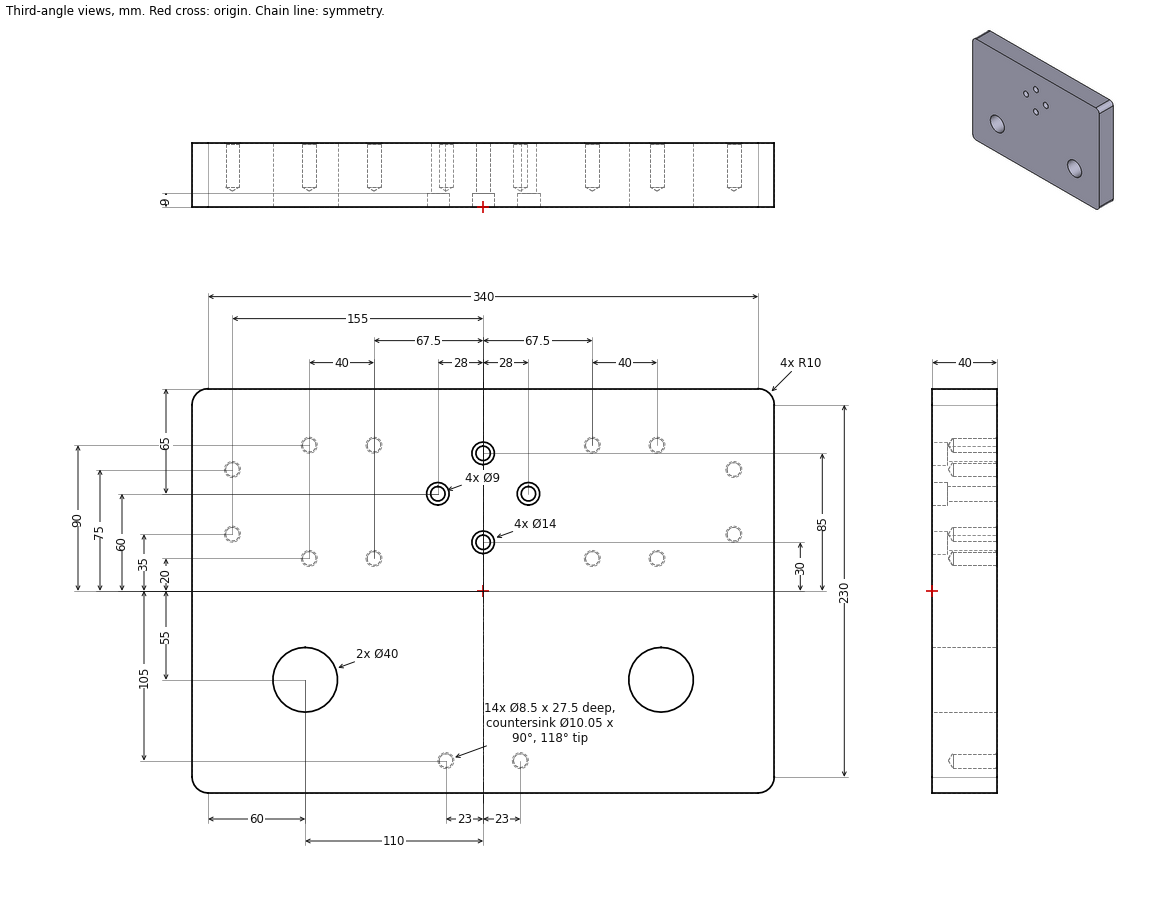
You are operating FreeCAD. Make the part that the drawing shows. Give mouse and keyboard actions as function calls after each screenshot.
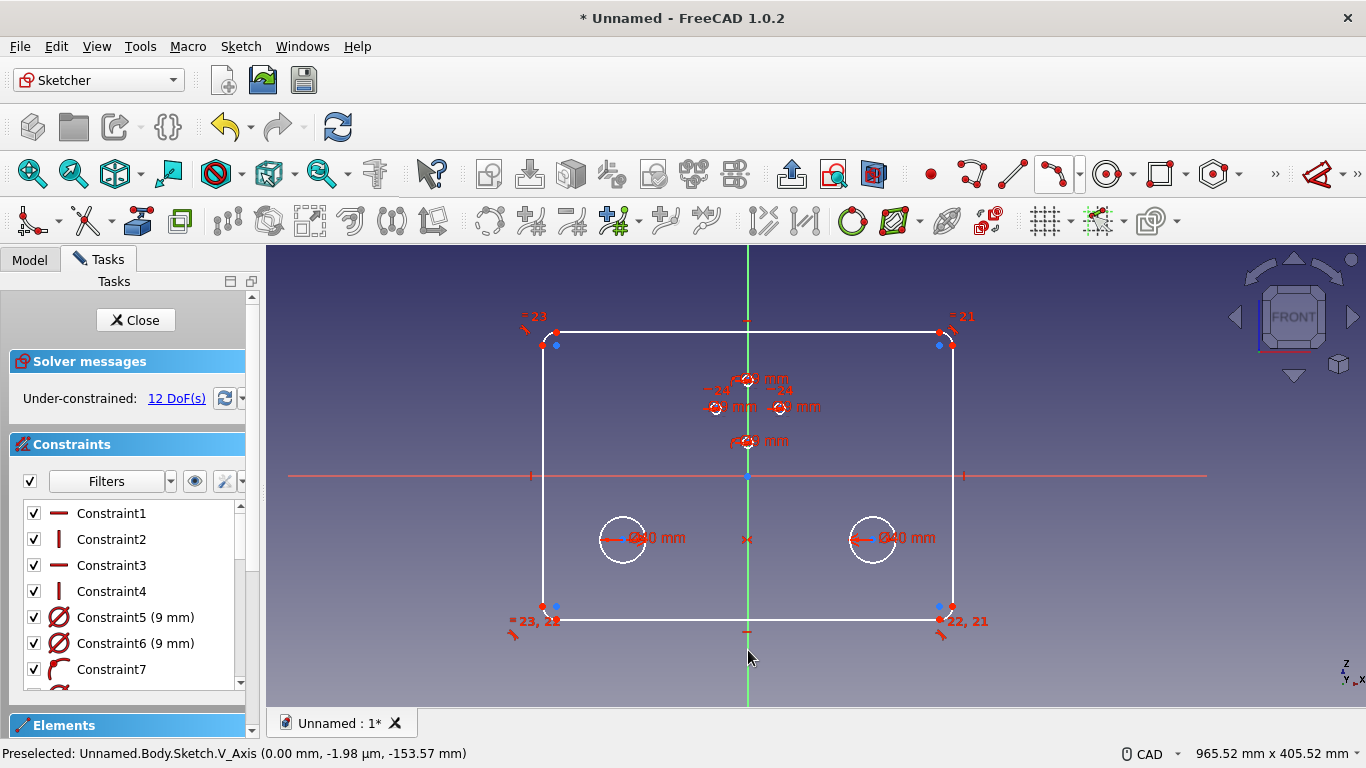
click(1316, 174)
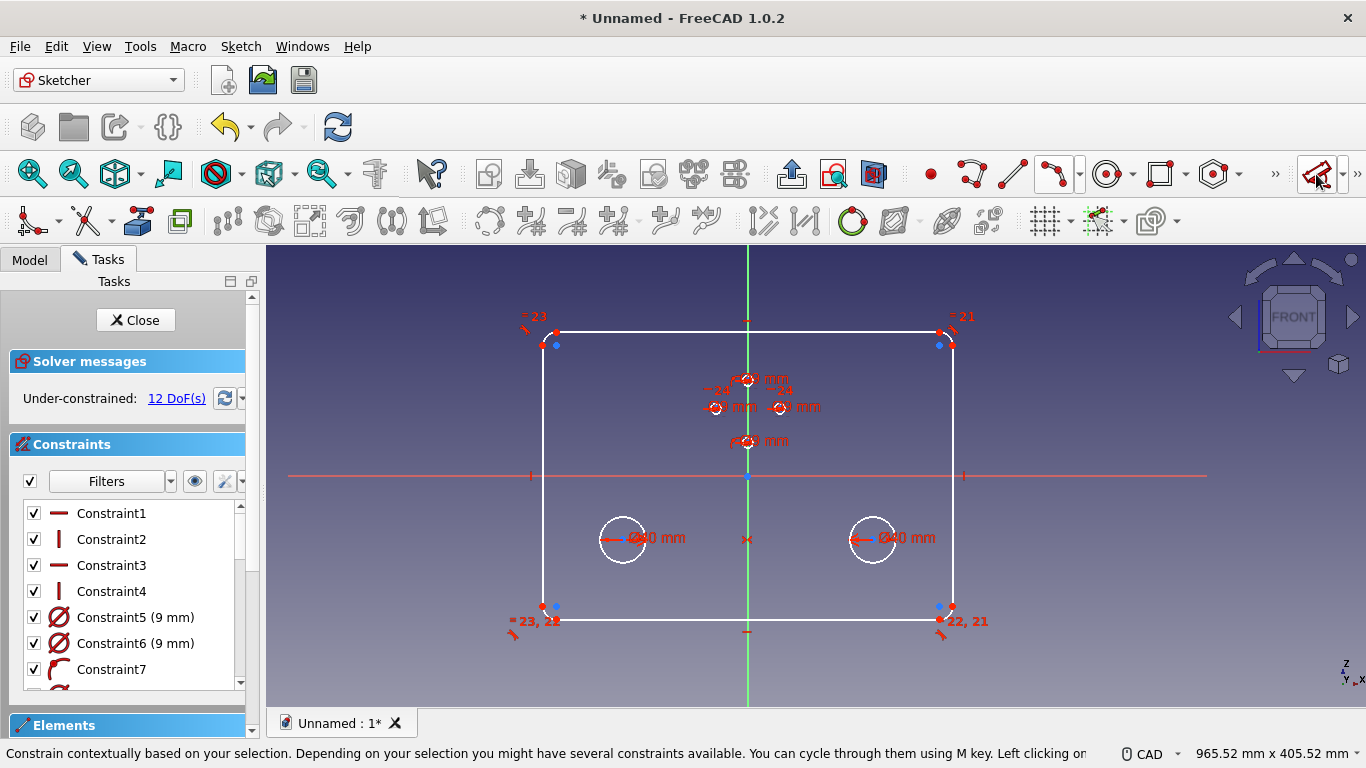
scroll(949, 336, up, 7)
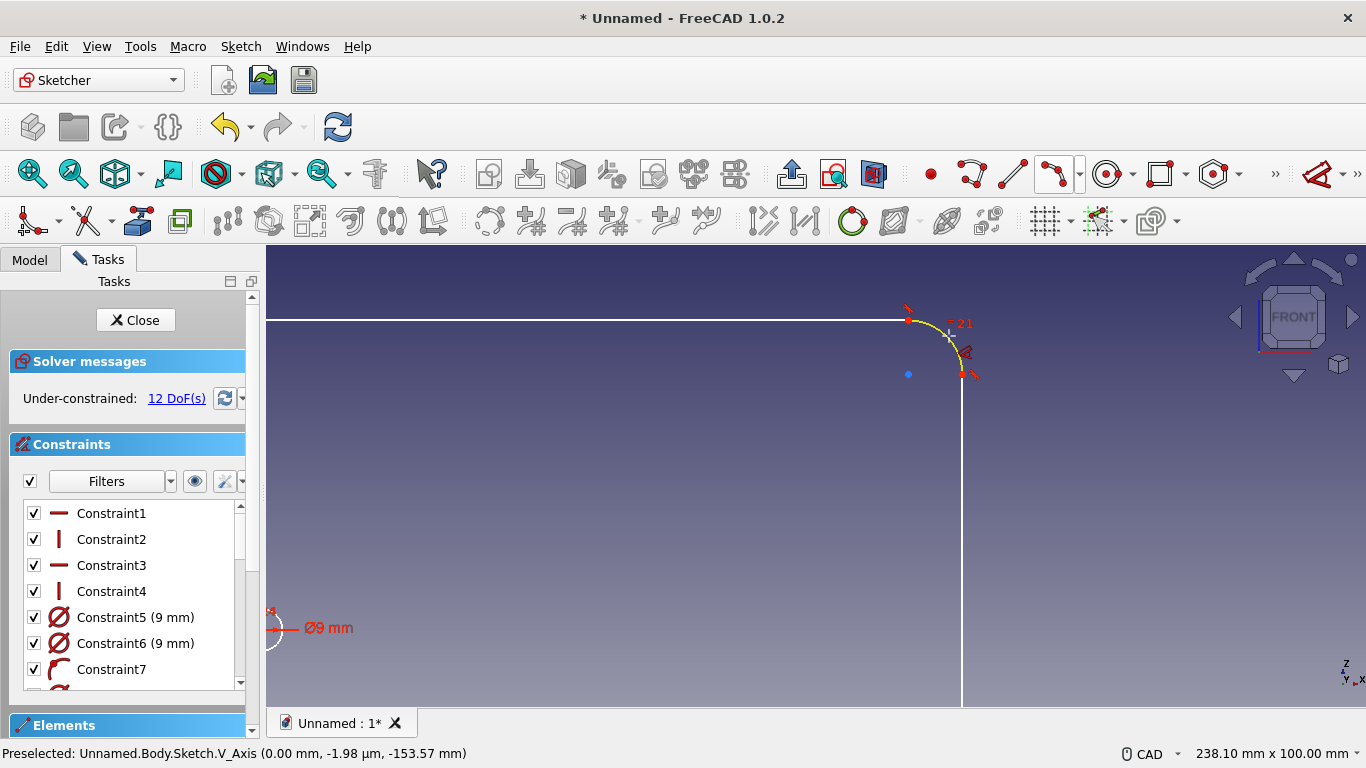
click(947, 336)
click(970, 313)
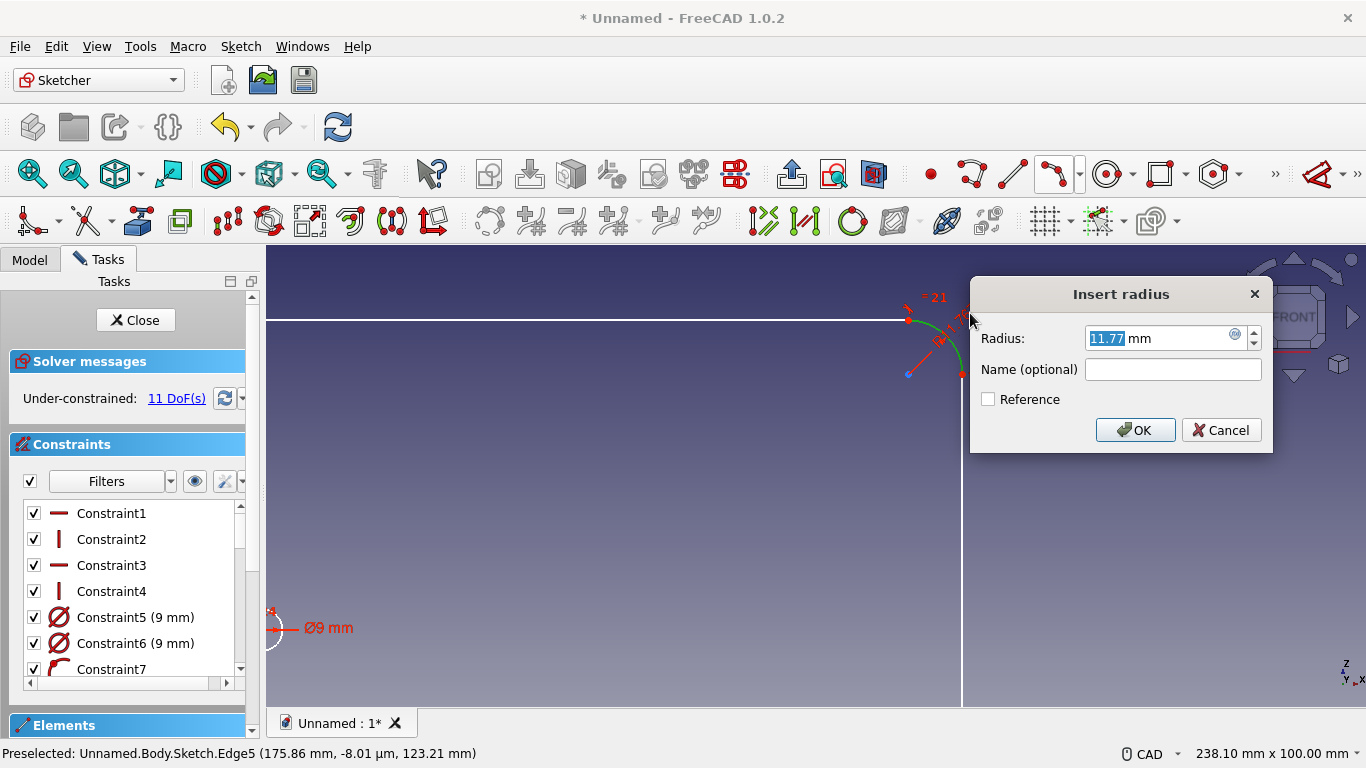
text(10)
key(Return)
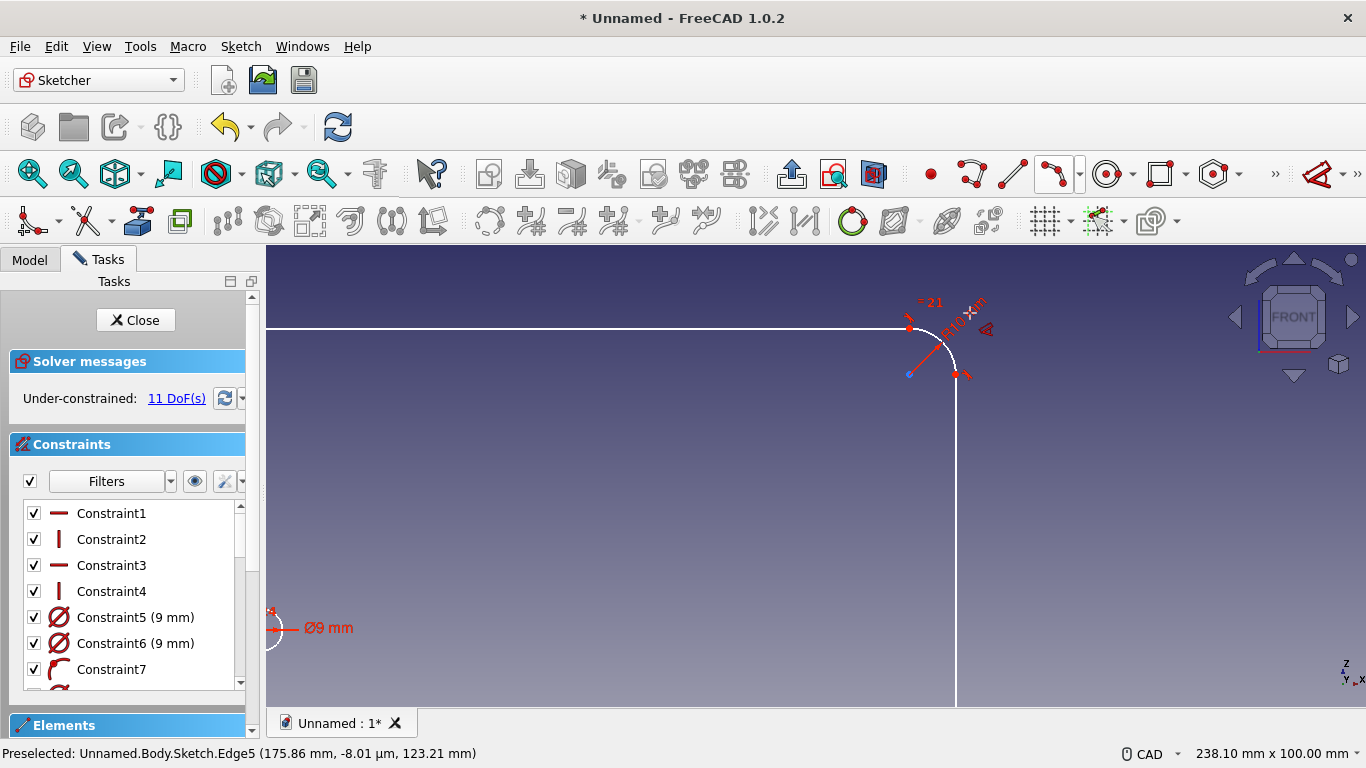
scroll(949, 336, down, 7)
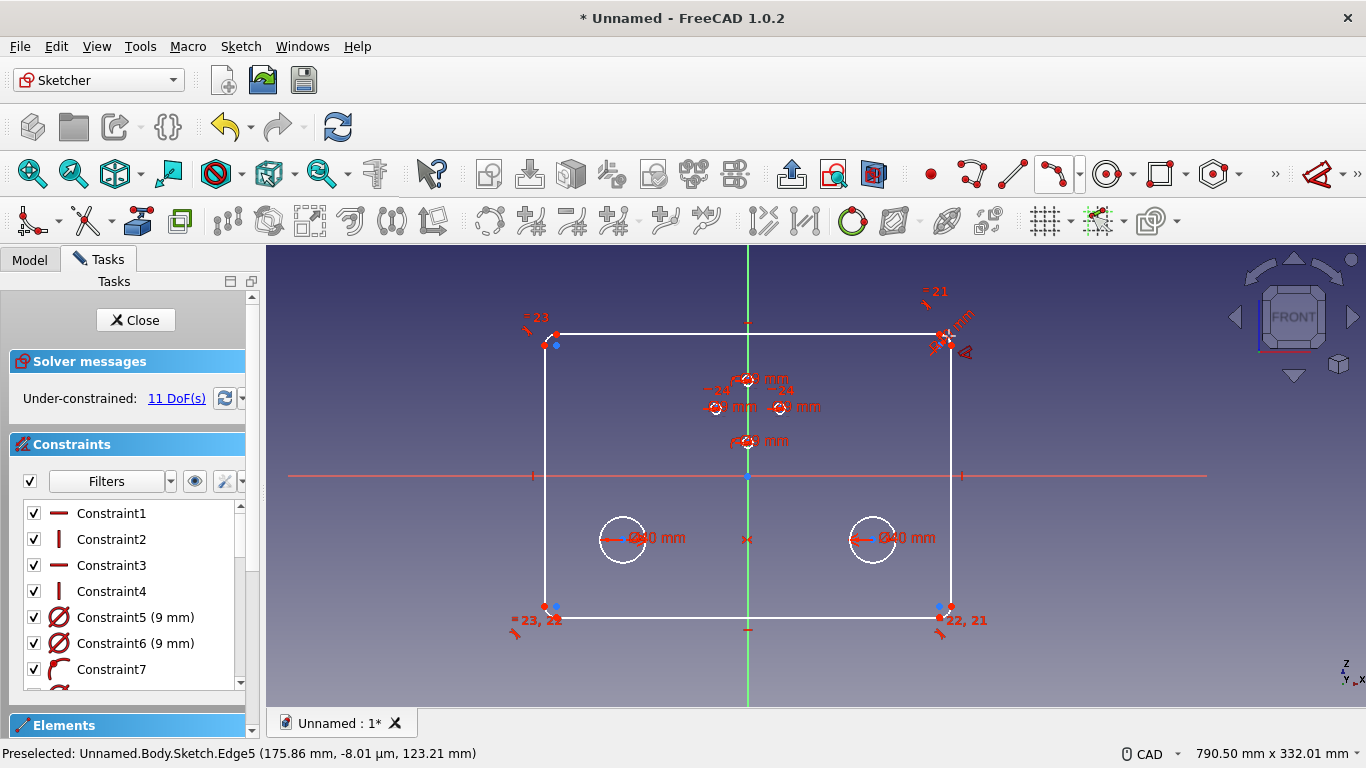
scroll(716, 409, up, 2)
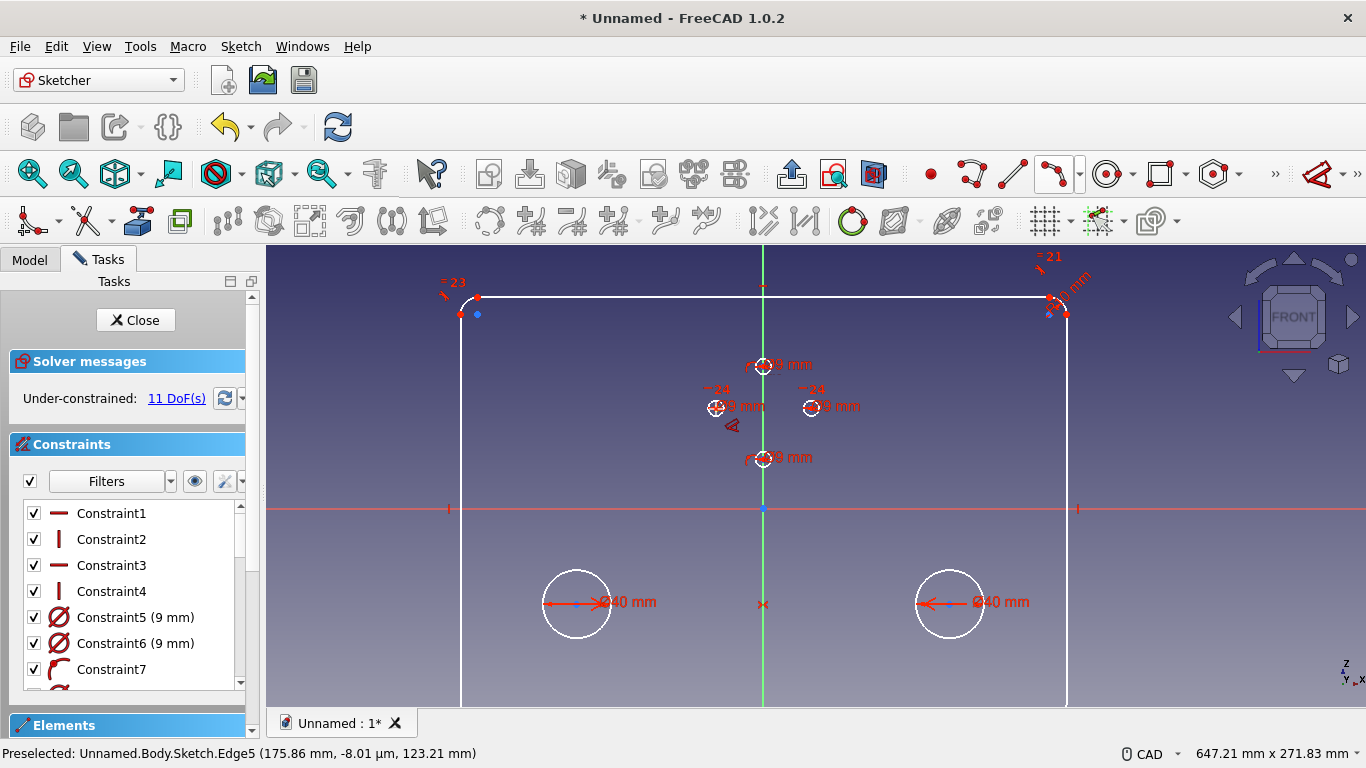
click(716, 408)
click(740, 374)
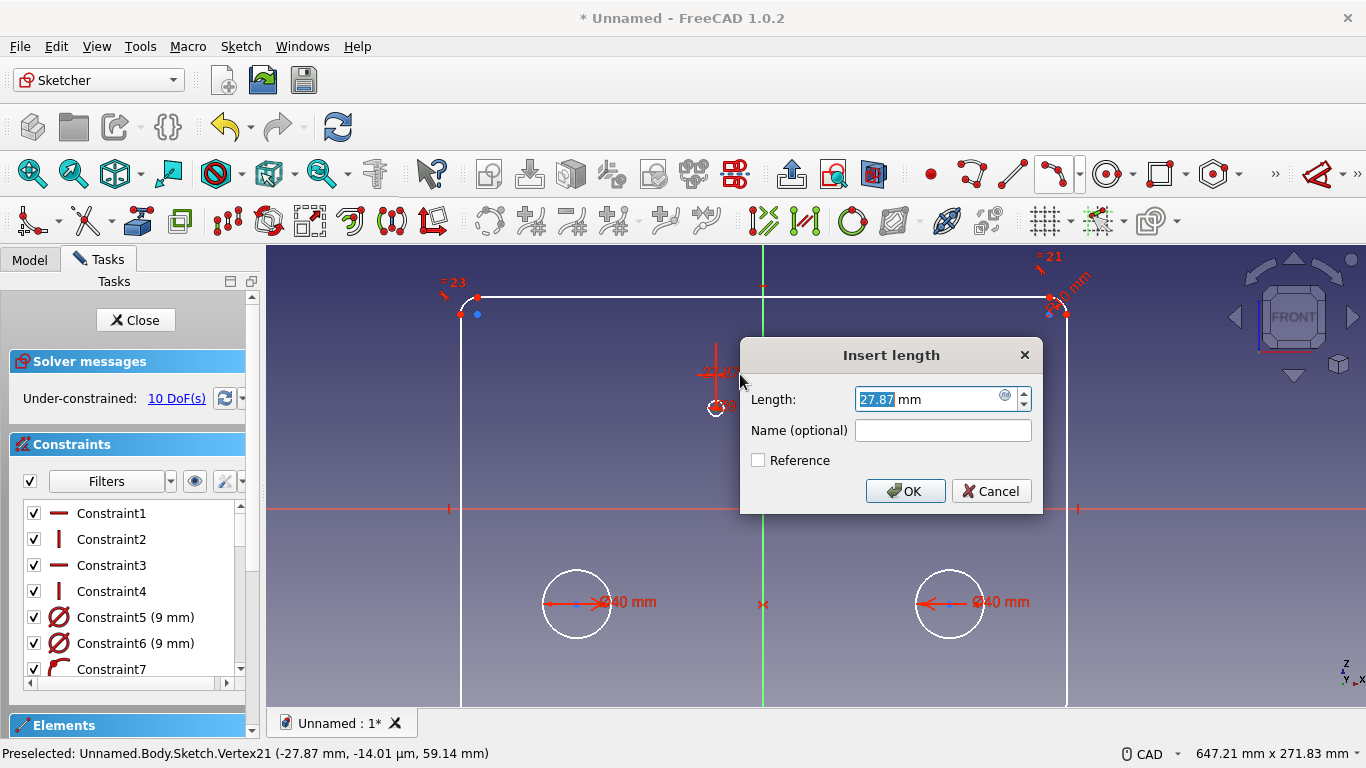
text(28)
key(Return)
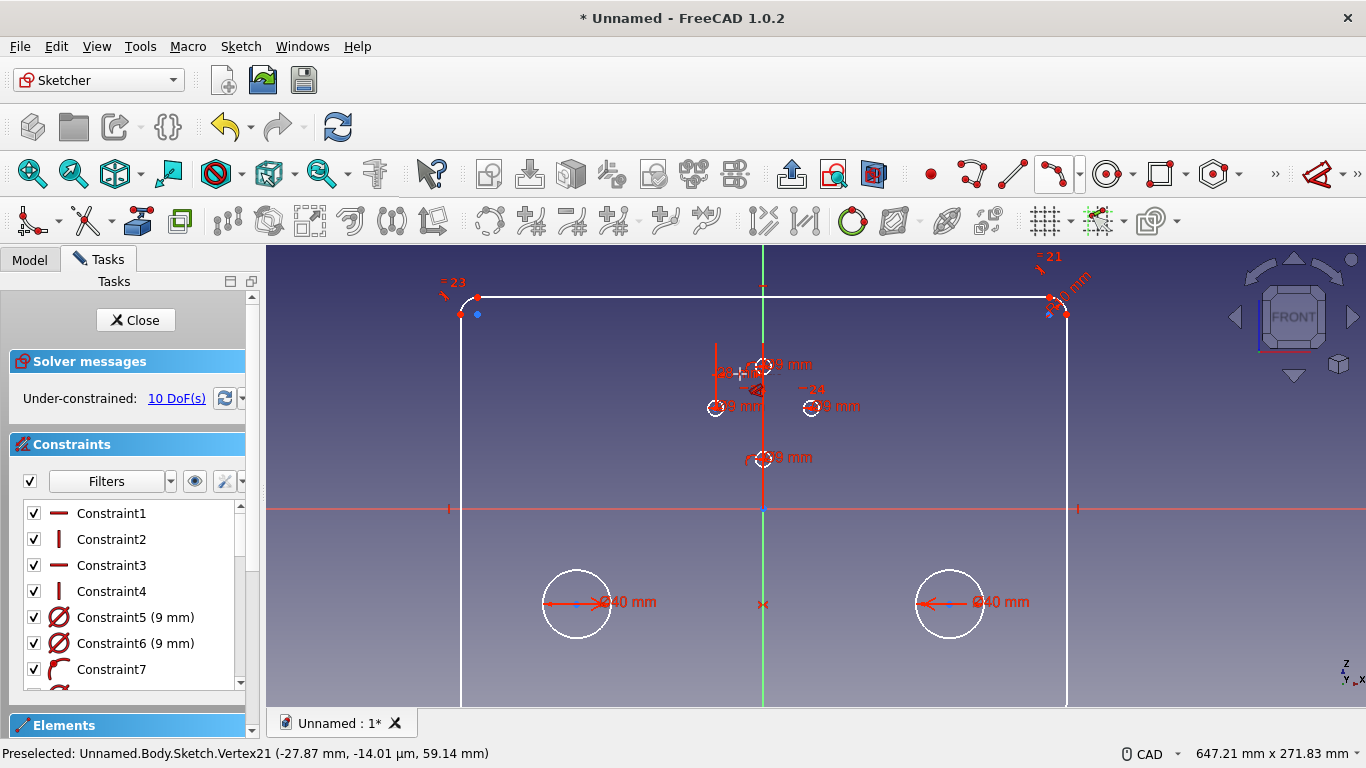
click(716, 408)
click(682, 459)